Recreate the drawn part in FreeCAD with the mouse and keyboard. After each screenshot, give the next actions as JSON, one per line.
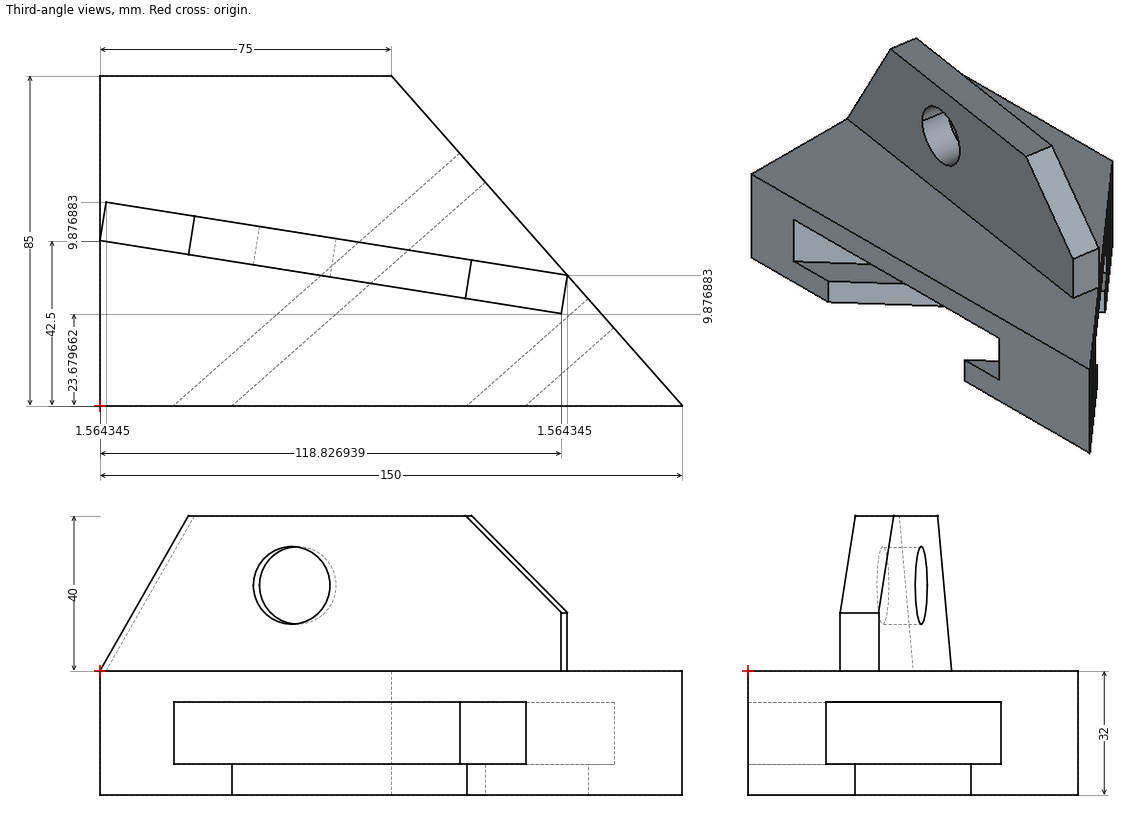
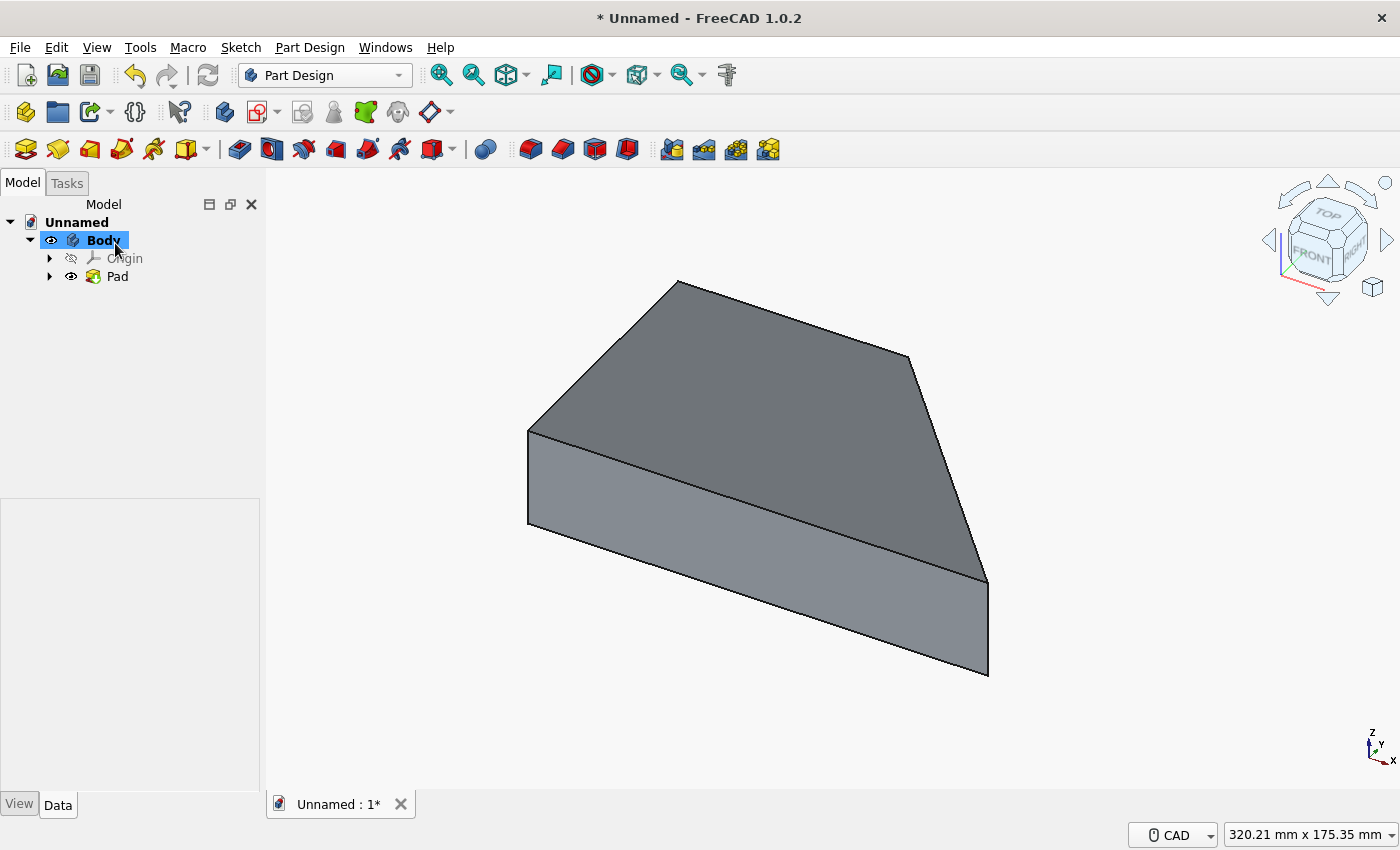
{"action": "key", "text": "3"}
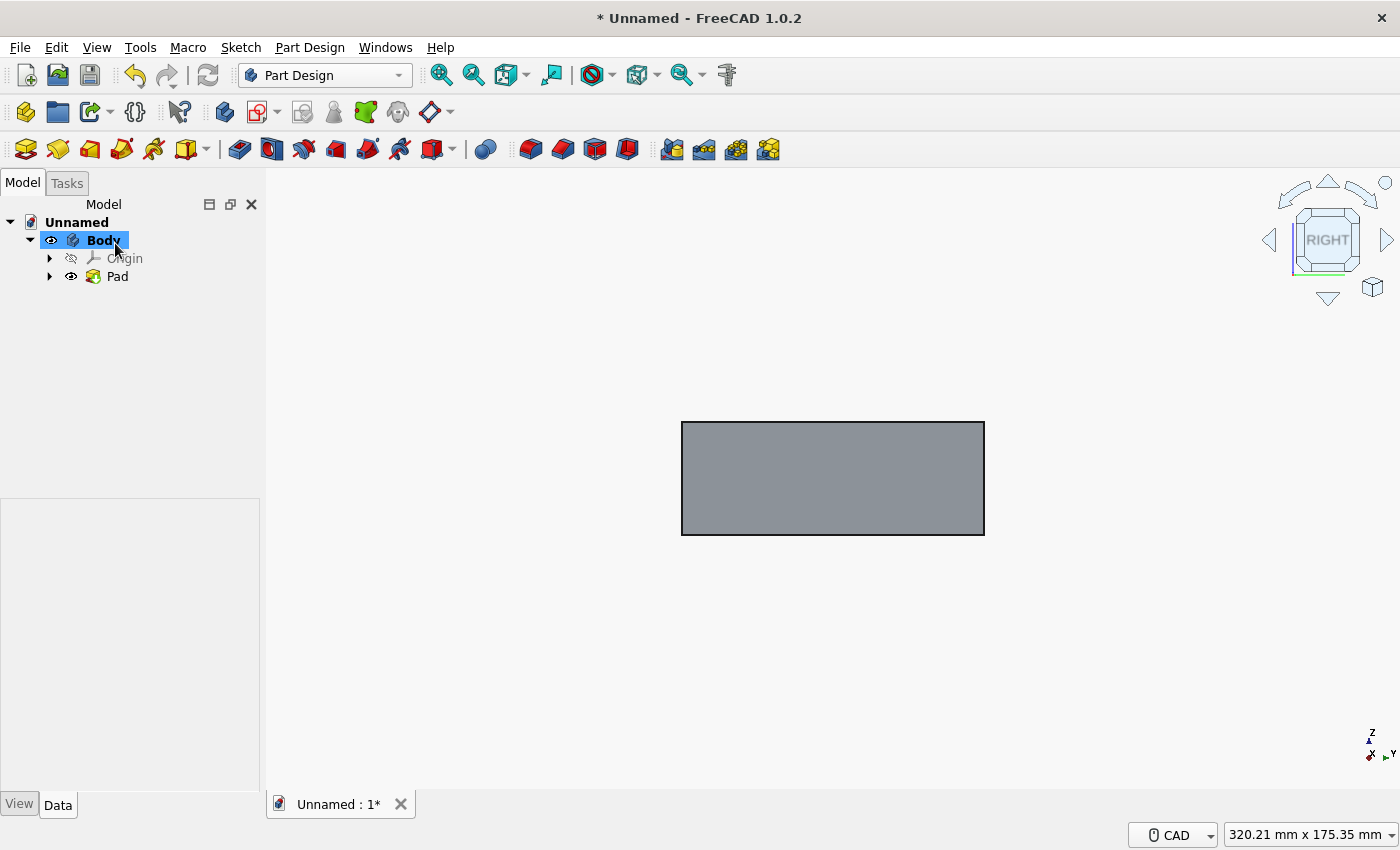
{"action": "key", "text": "v f"}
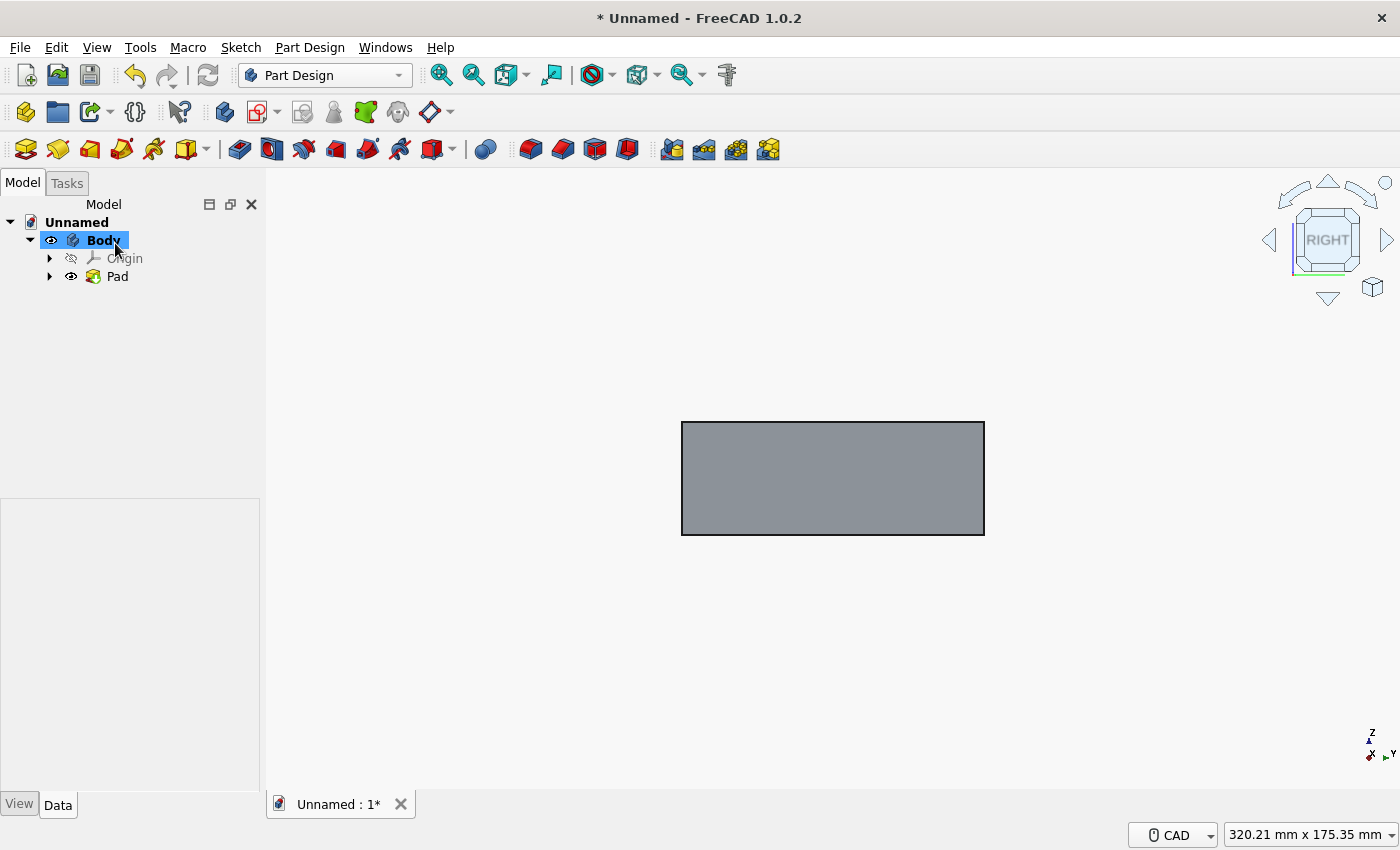
{"action": "left_click", "coordinate": [747, 477]}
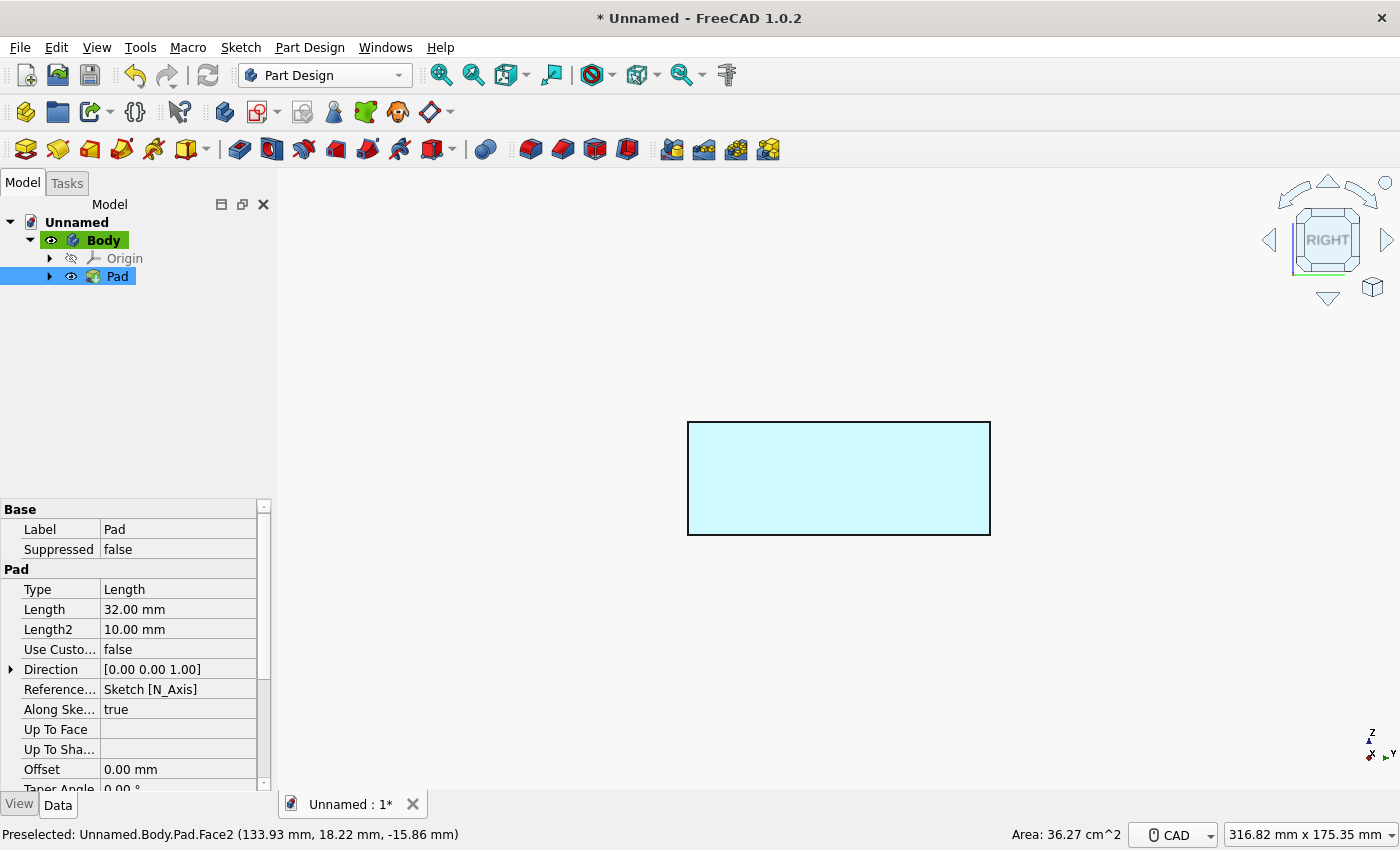
{"action": "left_click", "coordinate": [258, 112]}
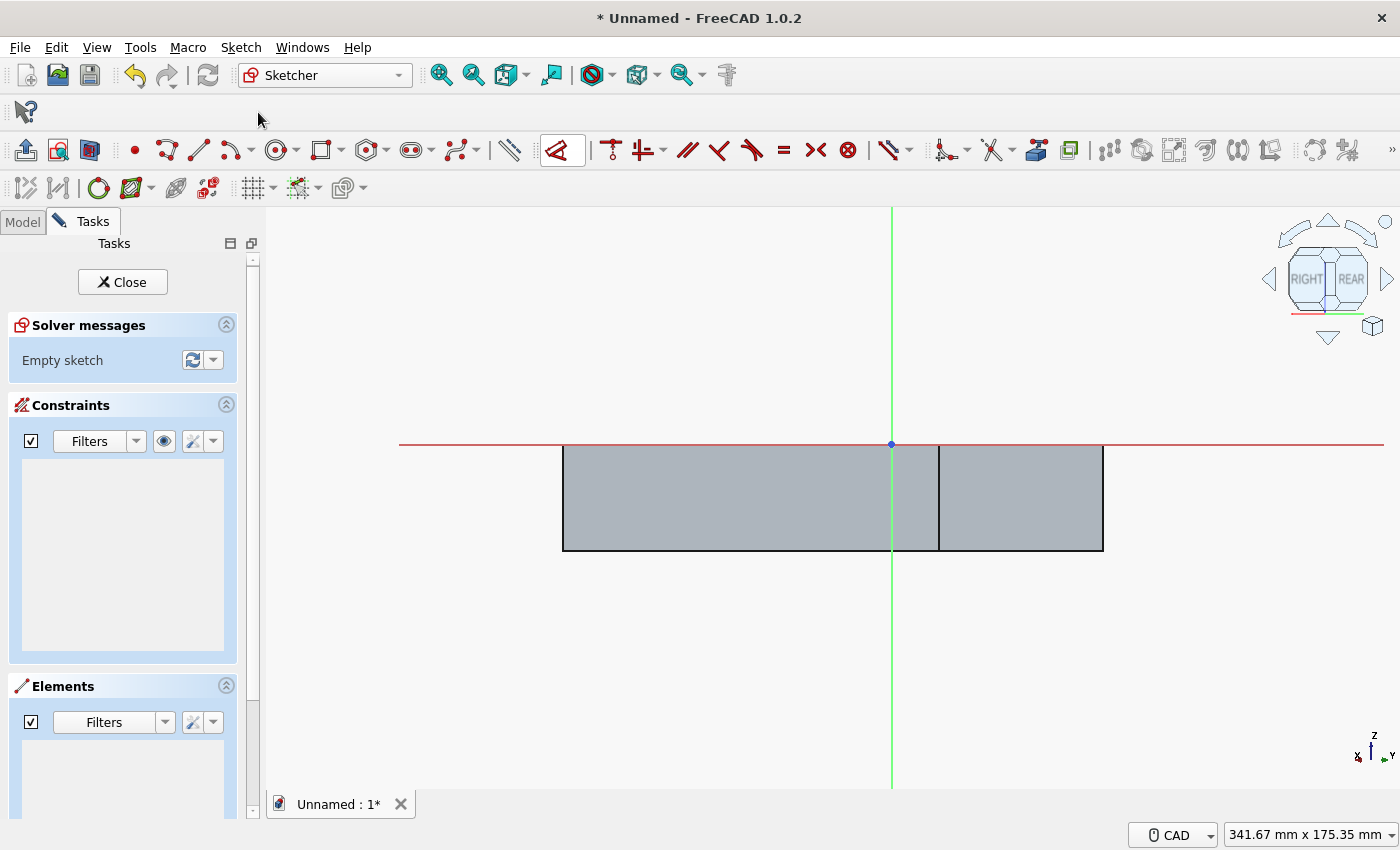
{"action": "scroll", "coordinate": [776, 498], "scroll_direction": "up", "scroll_amount": 5}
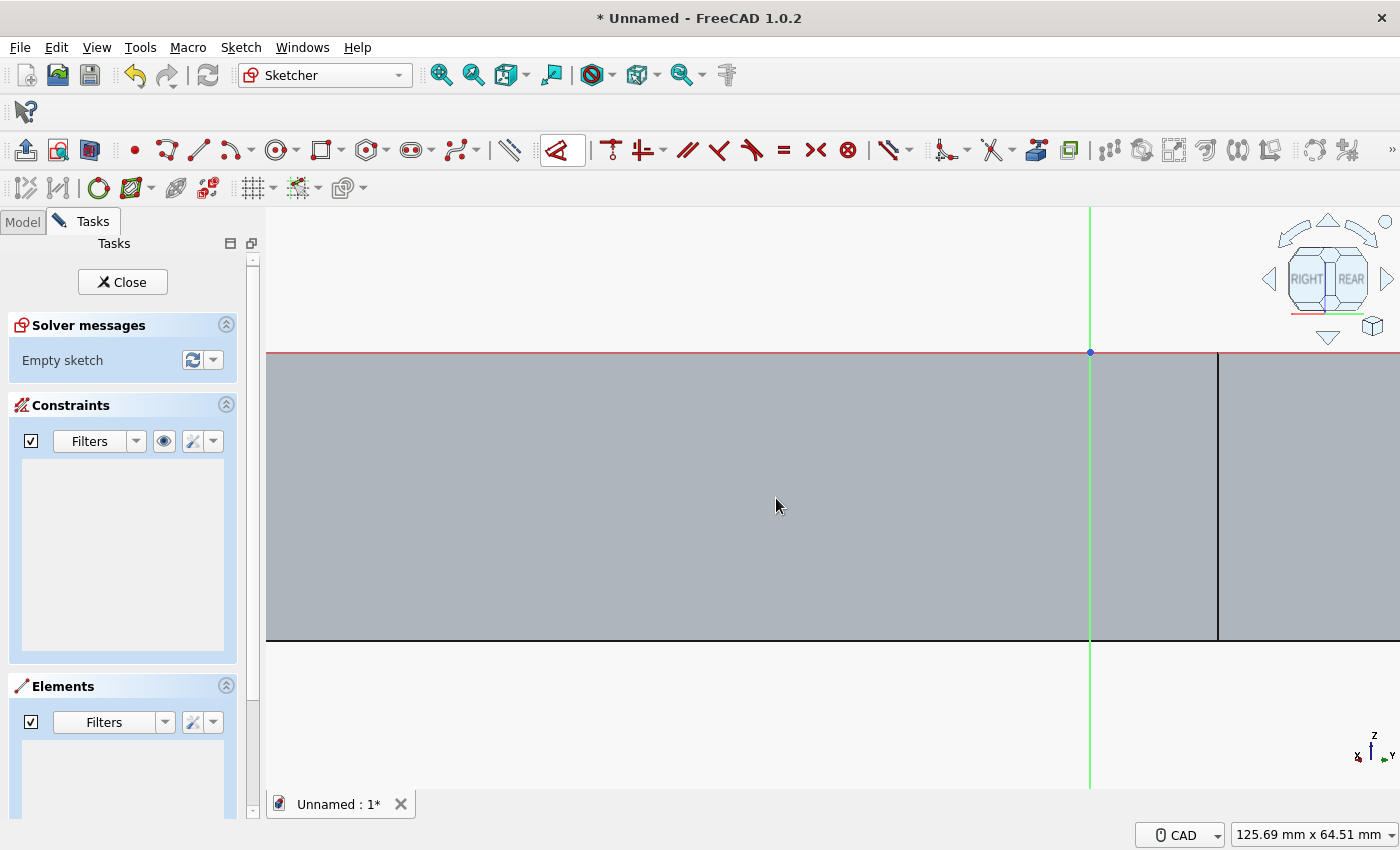
{"action": "key", "text": "g m"}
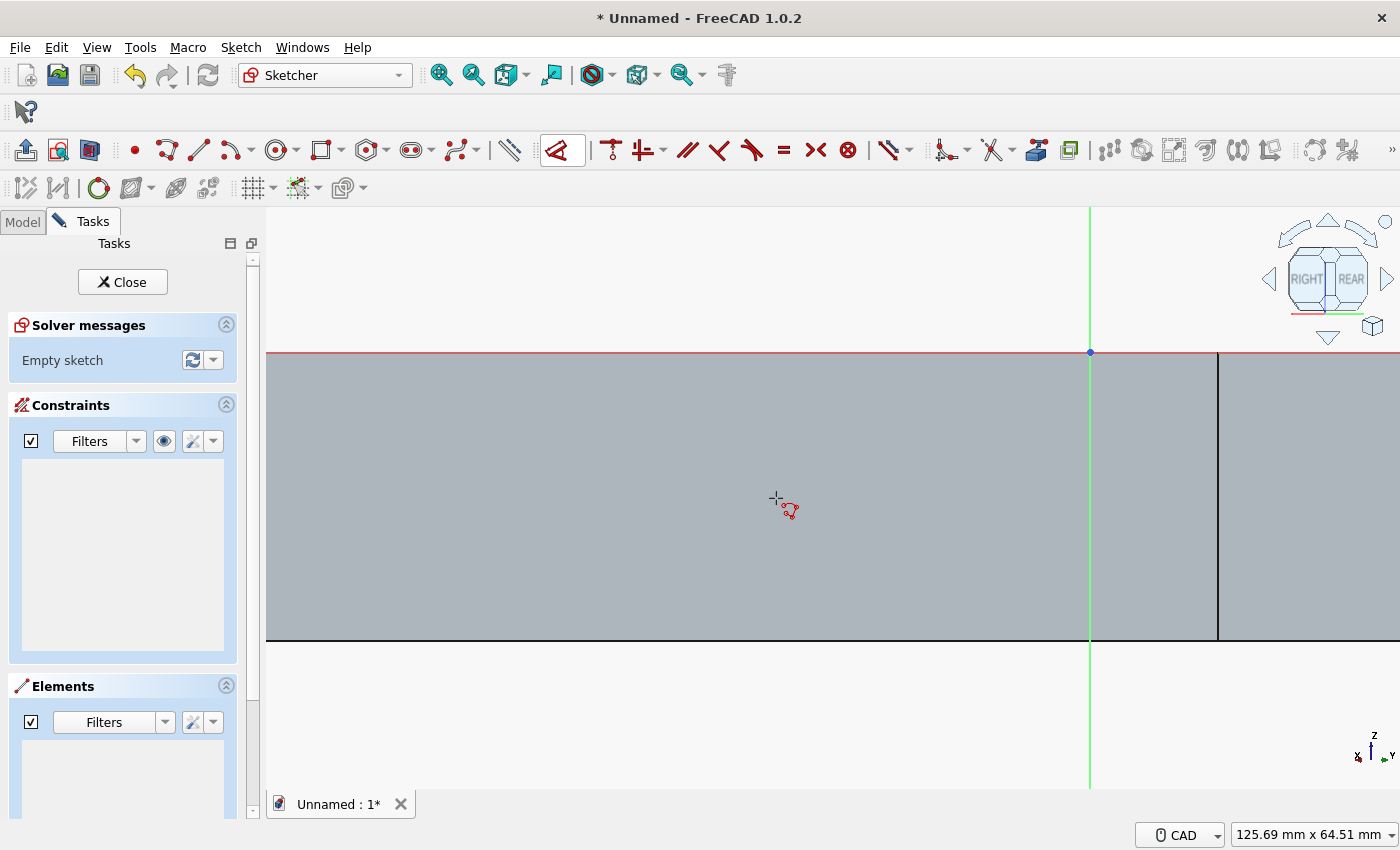
{"action": "left_click", "coordinate": [977, 425]}
{"action": "left_click", "coordinate": [436, 425]}
{"action": "left_click", "coordinate": [436, 569]}
{"action": "left_click", "coordinate": [526, 569]}
{"action": "left_click", "coordinate": [526, 641]}
{"action": "left_click", "coordinate": [887, 641]}
{"action": "left_click", "coordinate": [887, 569]}
{"action": "left_click", "coordinate": [977, 569]}
{"action": "left_click", "coordinate": [977, 426]}
{"action": "key", "text": "Escape"}
{"action": "key", "text": "Escape"}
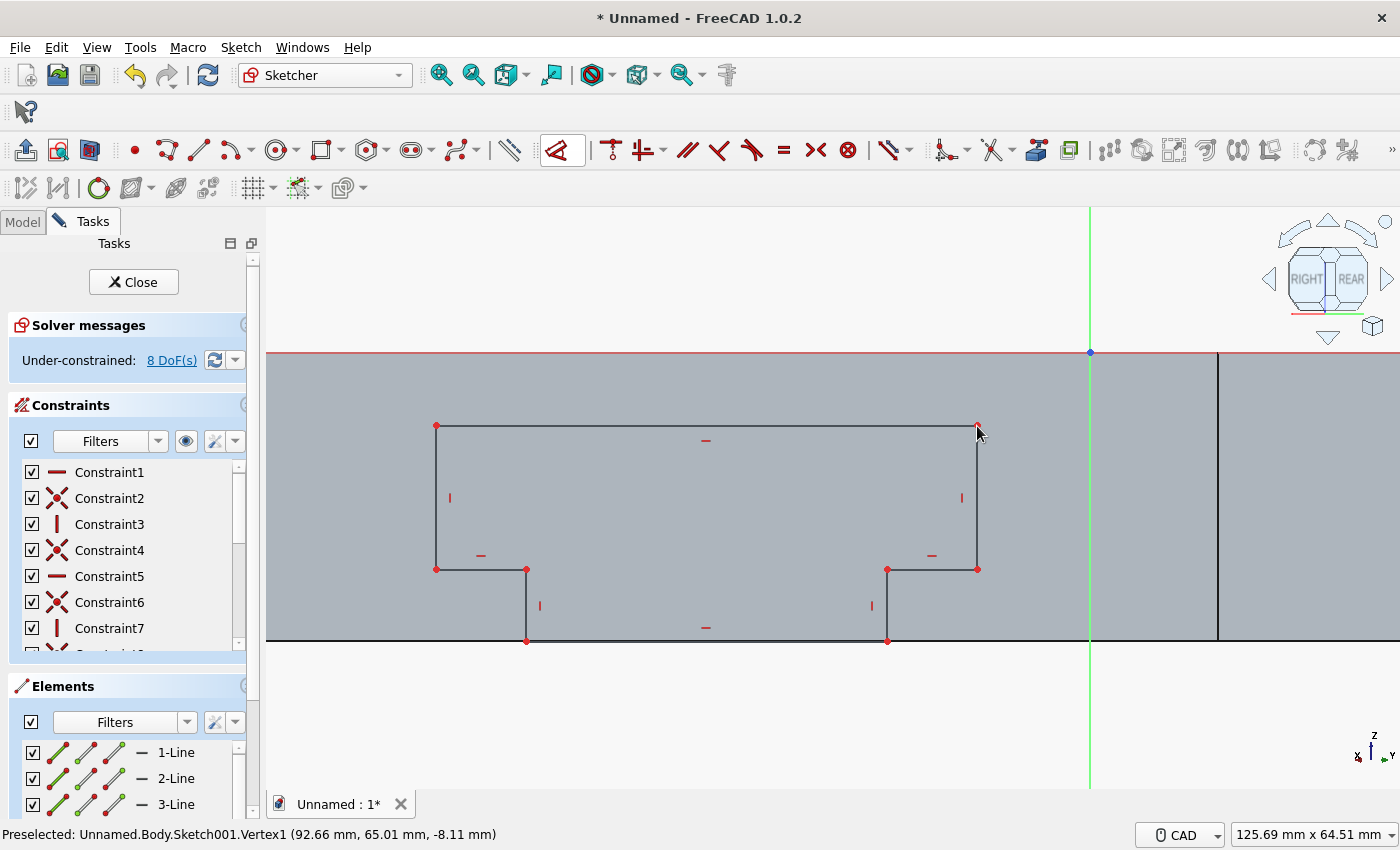
{"action": "left_click", "coordinate": [526, 592]}